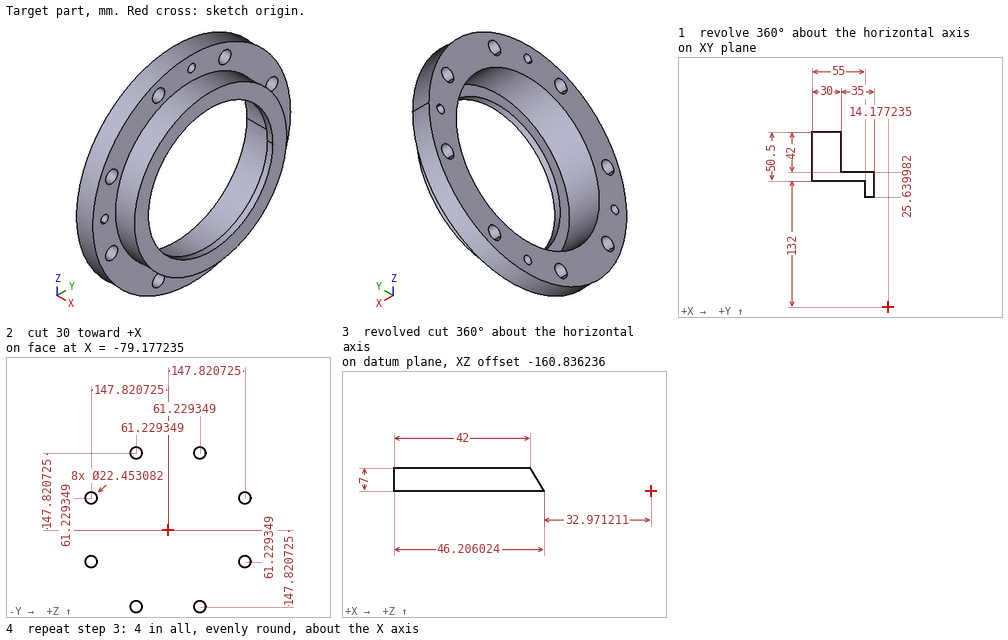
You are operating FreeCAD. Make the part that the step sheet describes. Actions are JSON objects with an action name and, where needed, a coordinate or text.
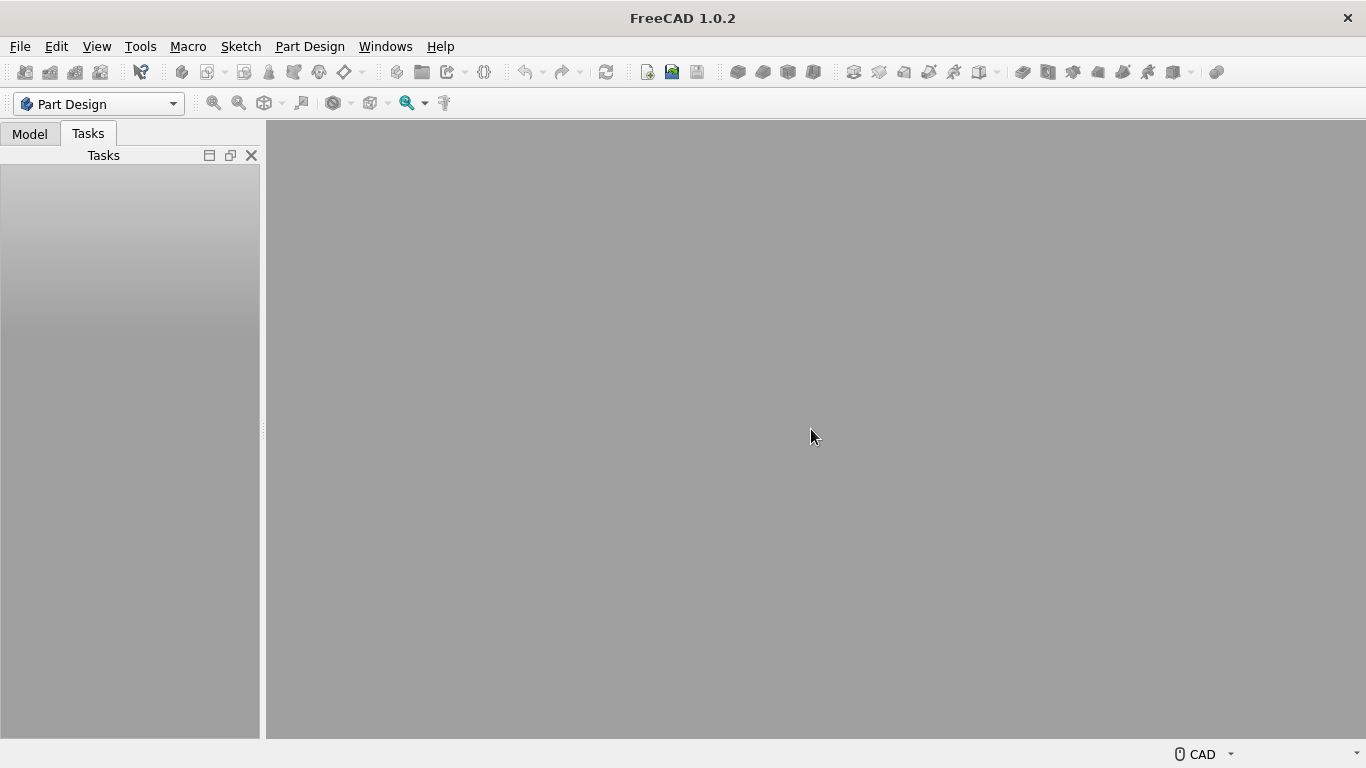
{"action": "left_click", "coordinate": [647, 72]}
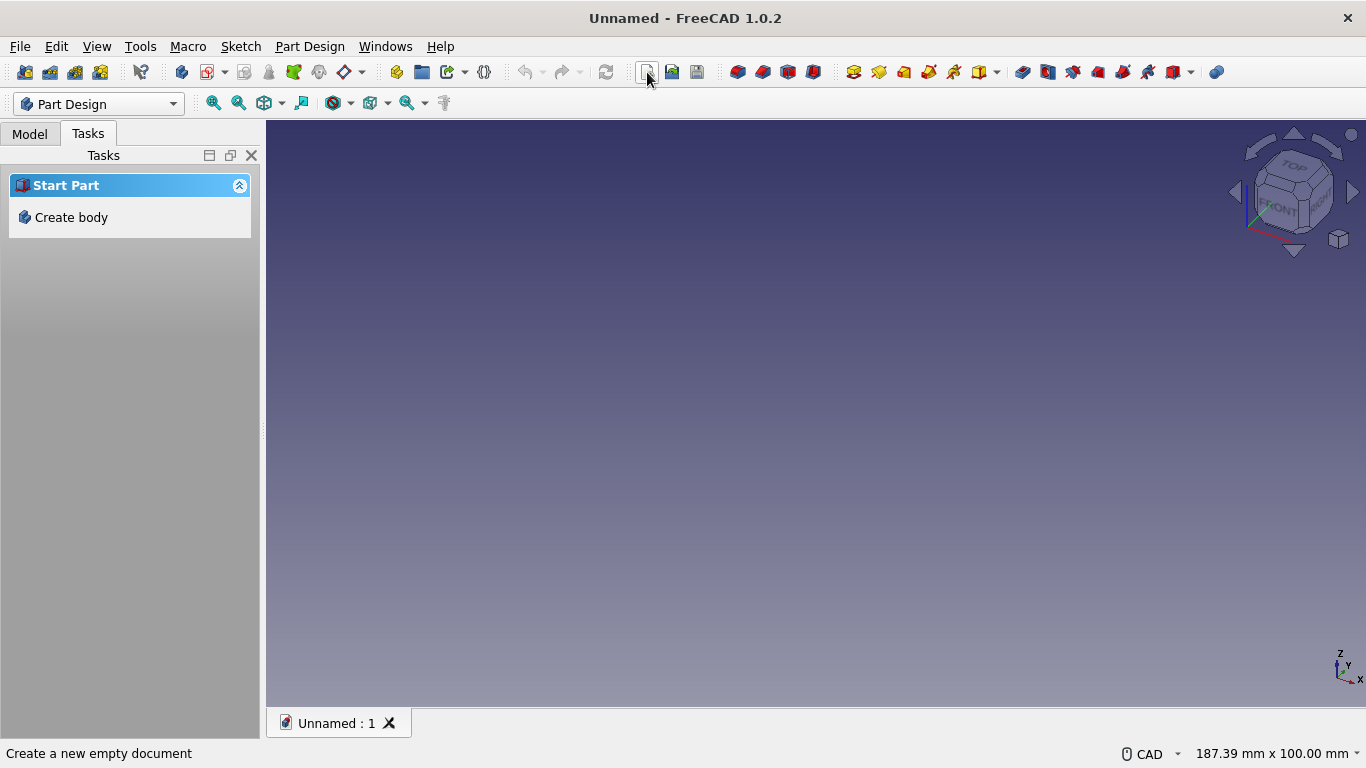
{"action": "left_click", "coordinate": [206, 72]}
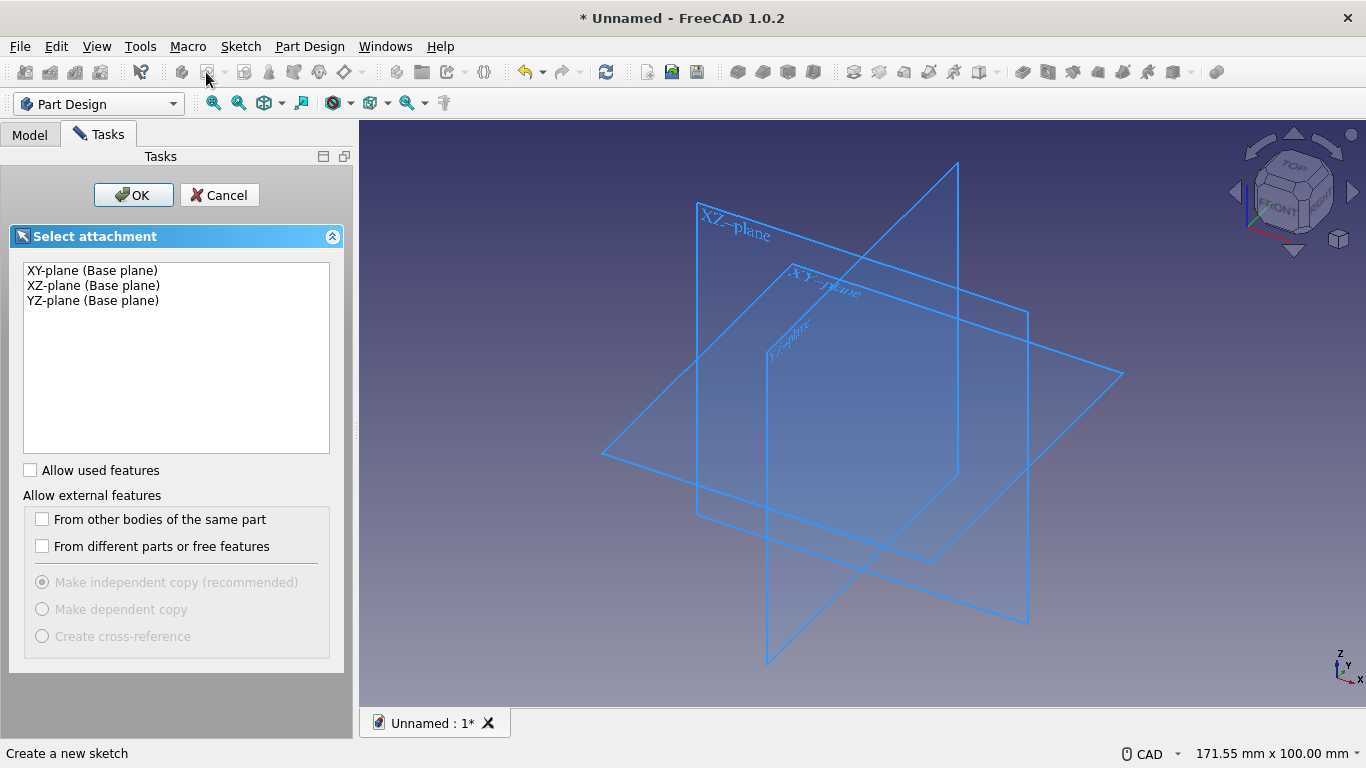
{"action": "left_click", "coordinate": [84, 270]}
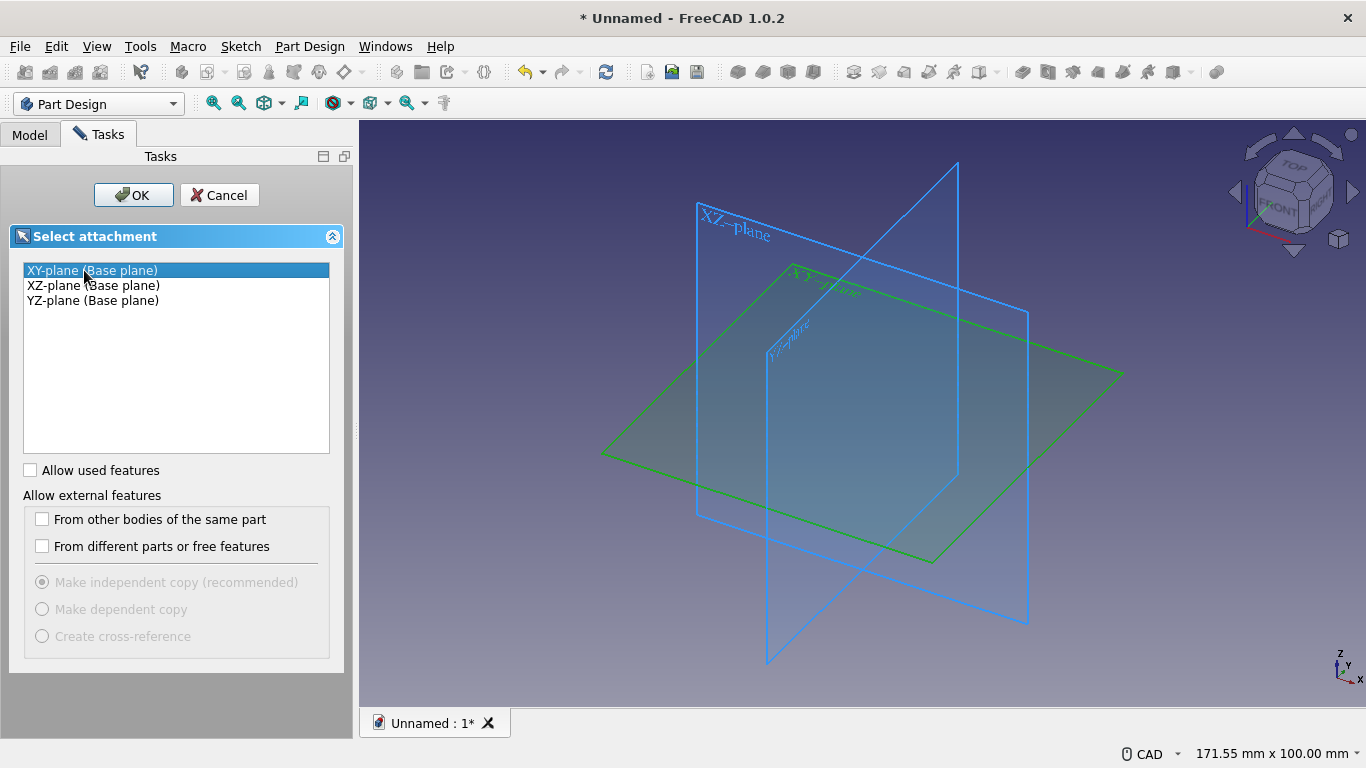
{"action": "left_click", "coordinate": [134, 195]}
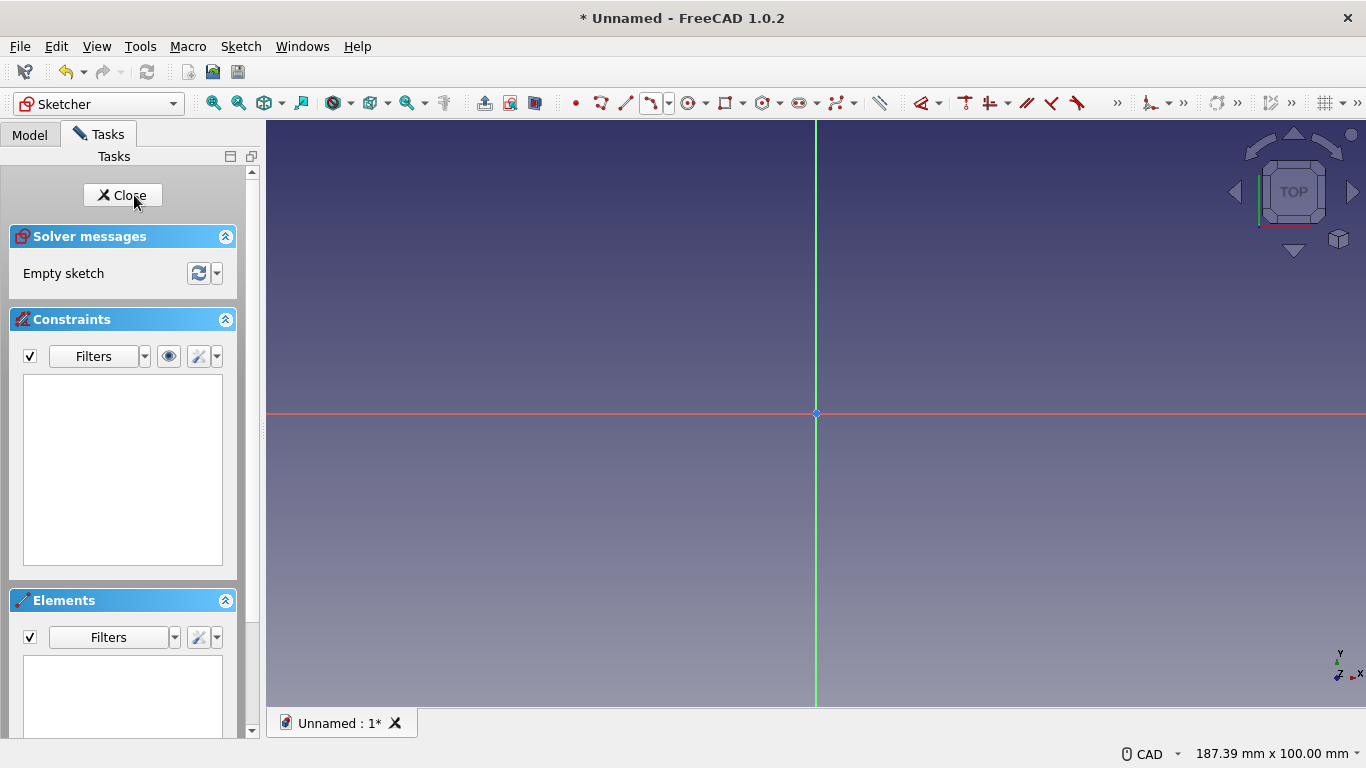
{"action": "scroll", "coordinate": [748, 414], "scroll_direction": "down", "scroll_amount": 5}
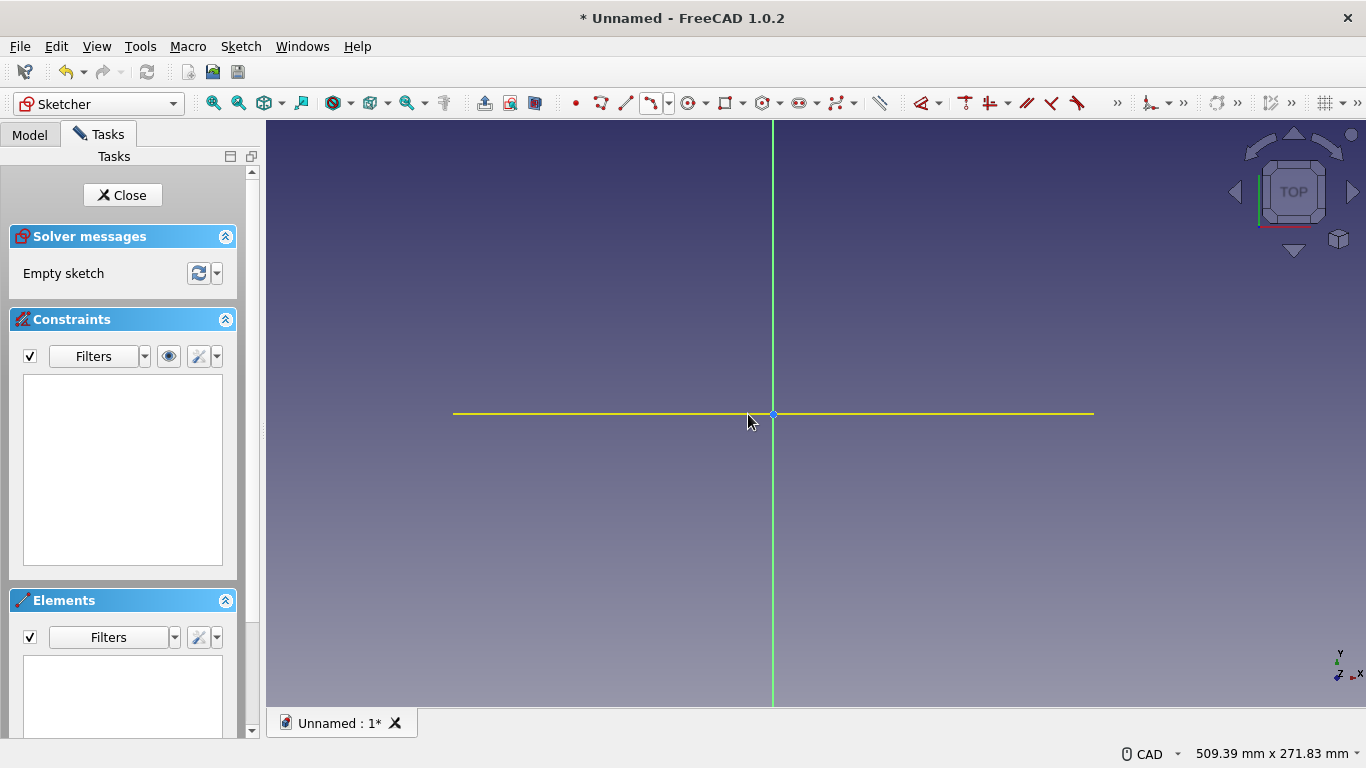
{"action": "scroll", "coordinate": [748, 414], "scroll_direction": "down", "scroll_amount": 5}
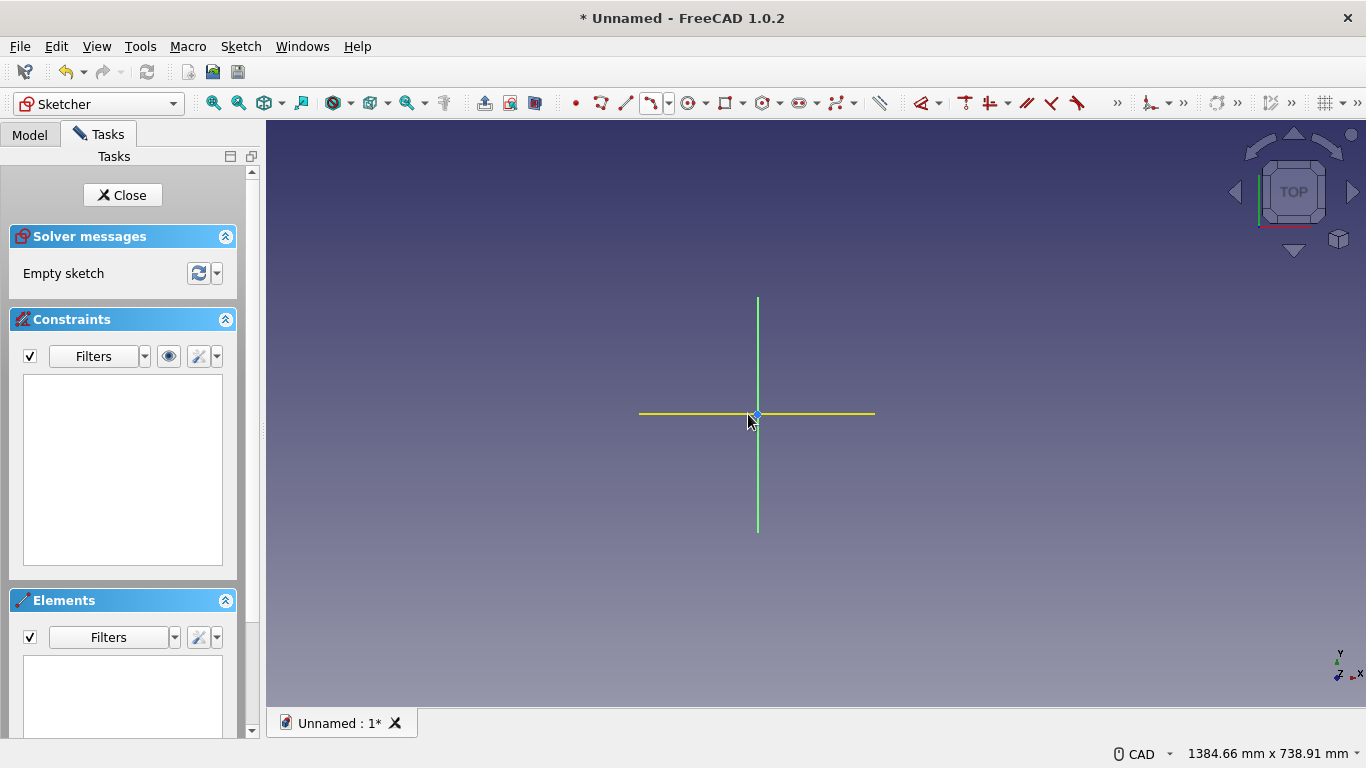
{"action": "scroll", "coordinate": [716, 278], "scroll_direction": "up", "scroll_amount": 10}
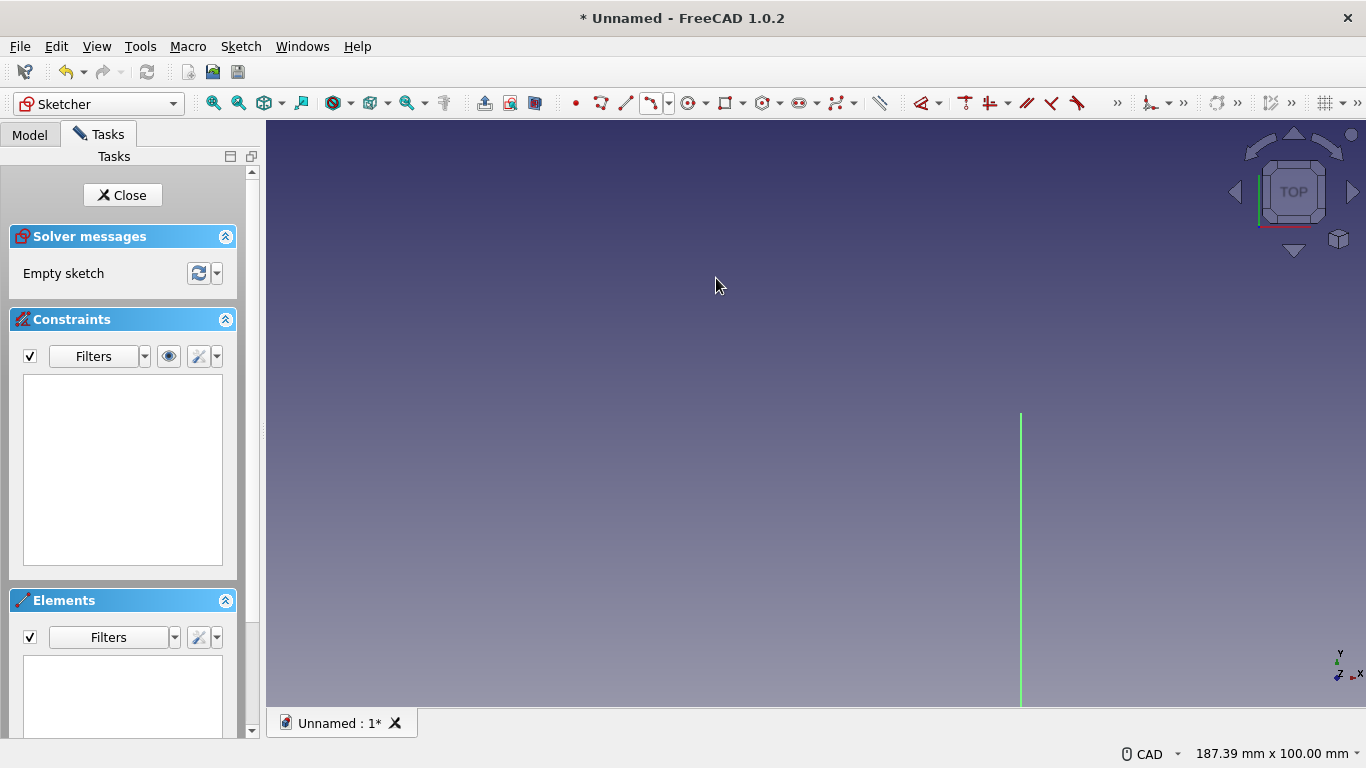
{"action": "left_click", "coordinate": [601, 104]}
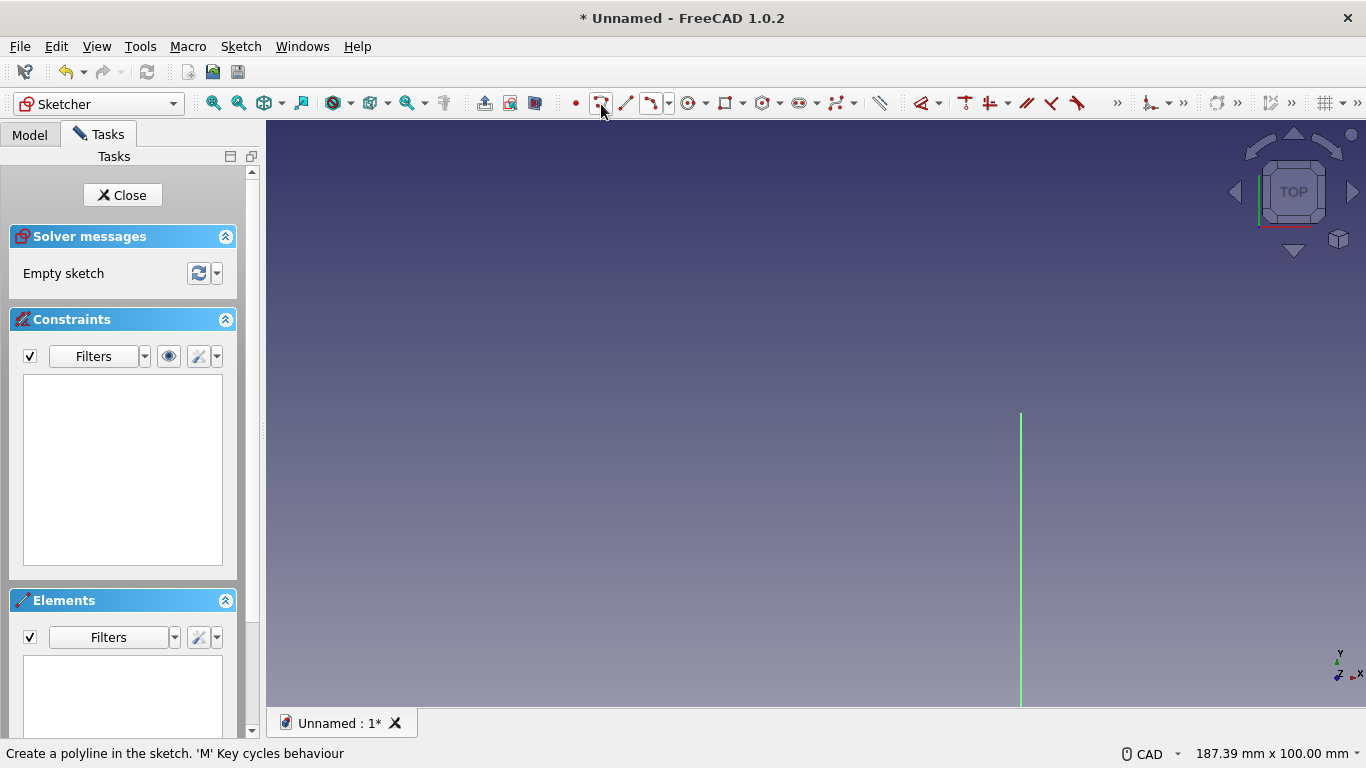
{"action": "left_click", "coordinate": [937, 610]}
{"action": "left_click", "coordinate": [937, 459]}
{"action": "left_click", "coordinate": [732, 459]}
{"action": "left_click", "coordinate": [732, 213]}
{"action": "left_click", "coordinate": [556, 213]}
{"action": "left_click", "coordinate": [556, 509]}
{"action": "left_click", "coordinate": [879, 509]}
{"action": "left_click", "coordinate": [879, 610]}
{"action": "left_click", "coordinate": [937, 611]}
{"action": "key", "text": "Escape"}
{"action": "key", "text": "Escape"}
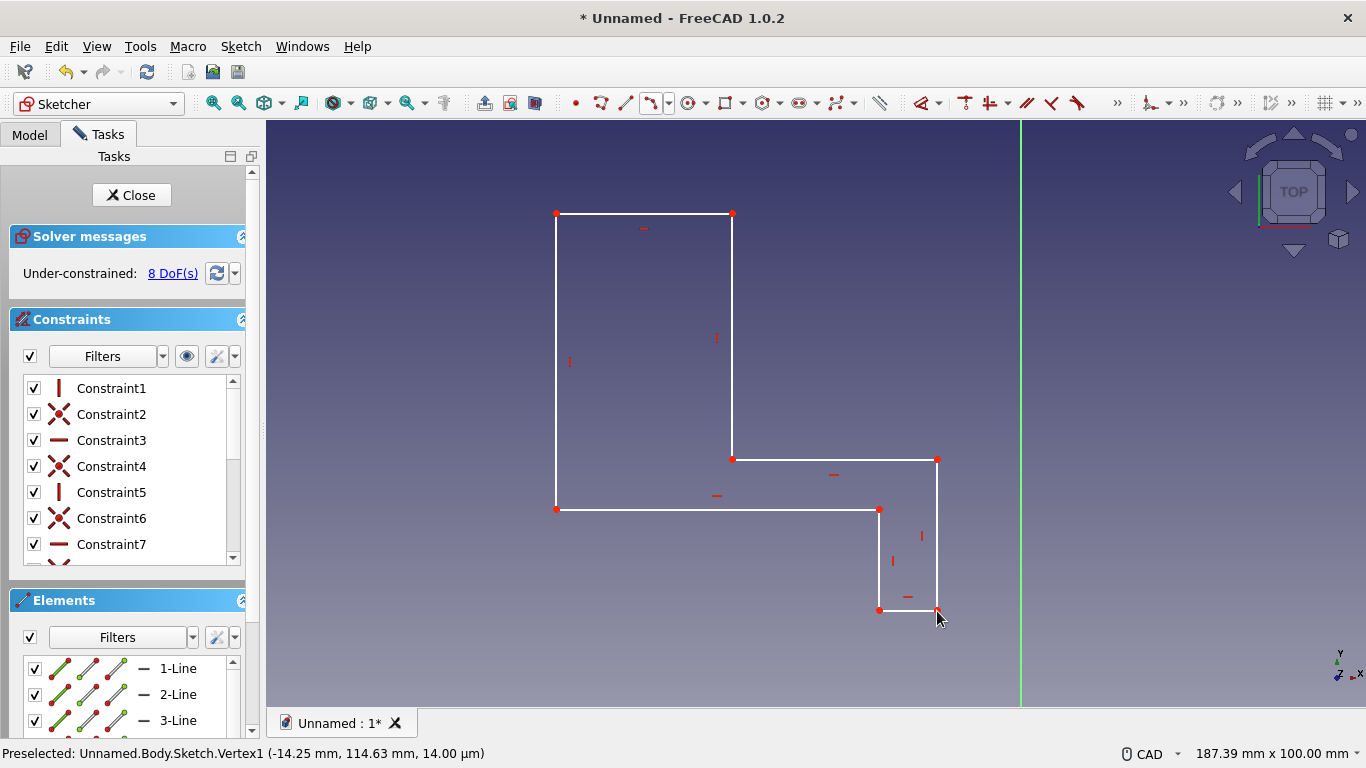
{"action": "left_click", "coordinate": [876, 460]}